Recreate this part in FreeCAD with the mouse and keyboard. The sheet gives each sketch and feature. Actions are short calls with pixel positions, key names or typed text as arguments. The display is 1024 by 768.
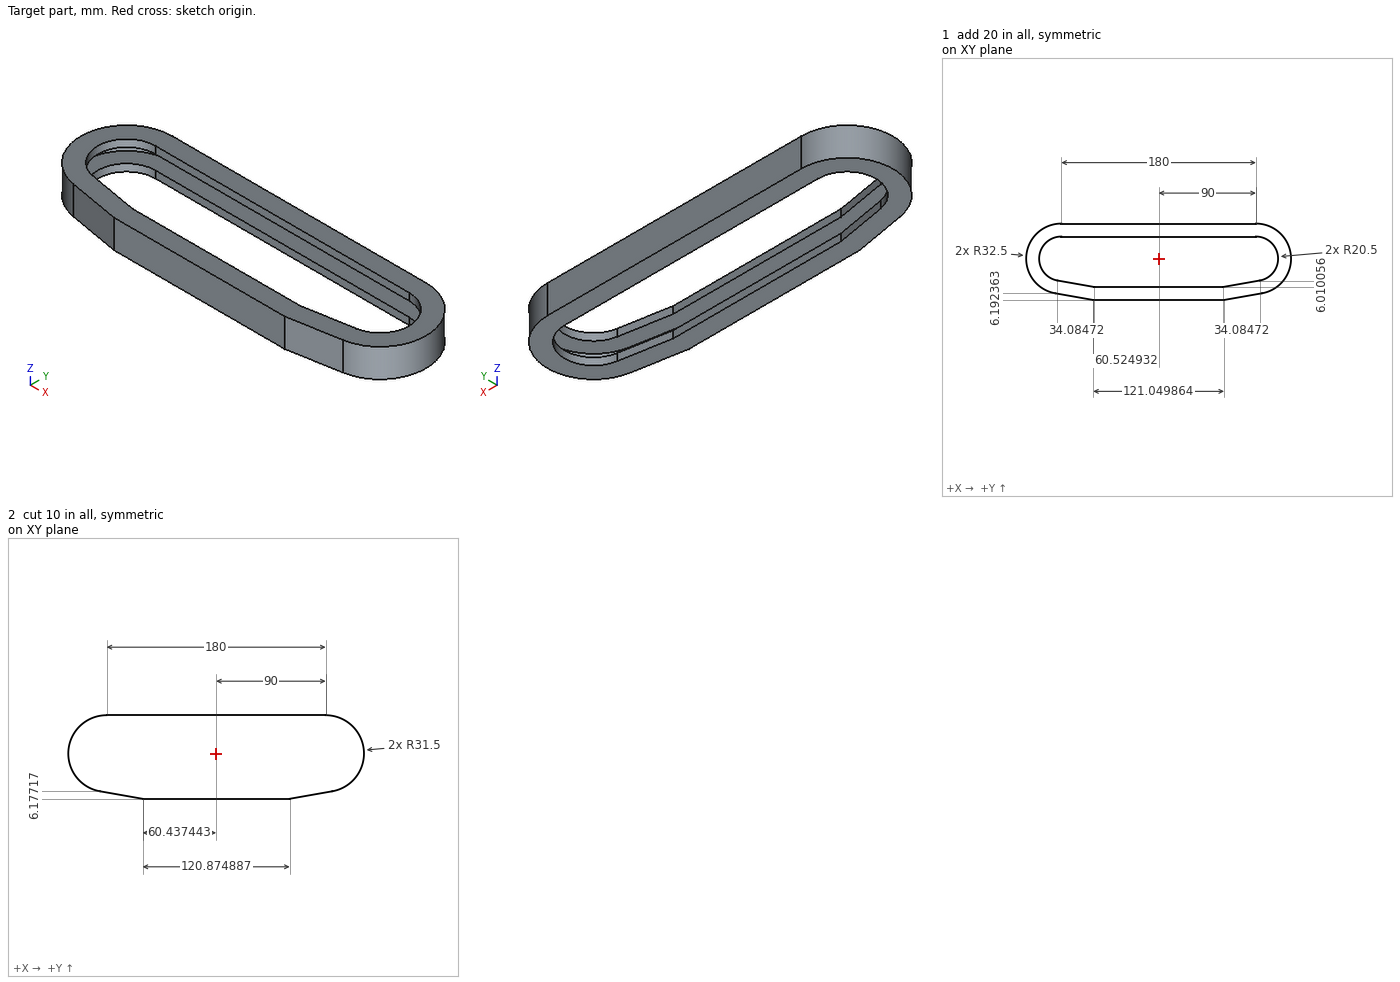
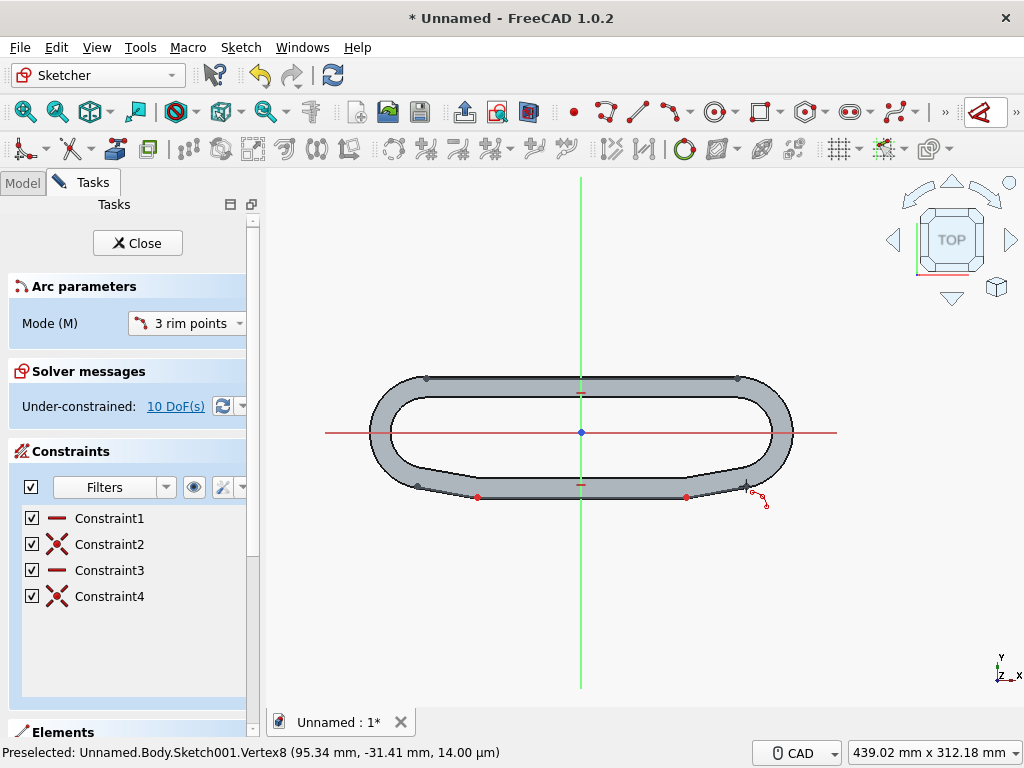
click(426, 379)
click(417, 487)
click(376, 412)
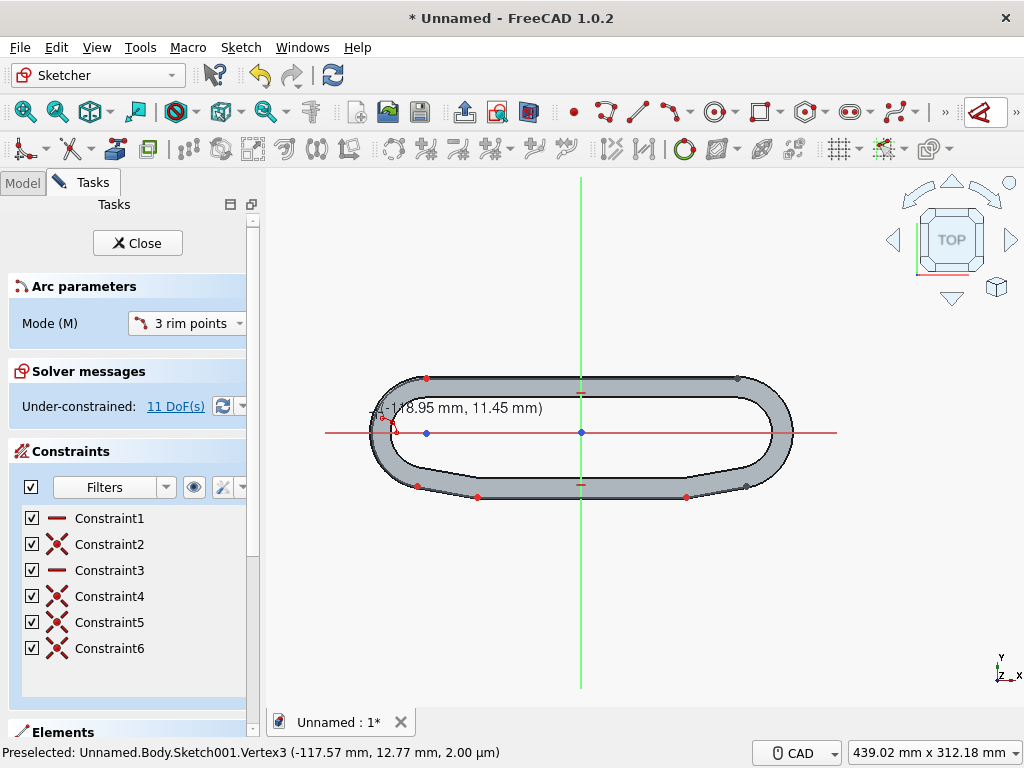
click(746, 487)
click(737, 379)
click(787, 412)
key(Escape)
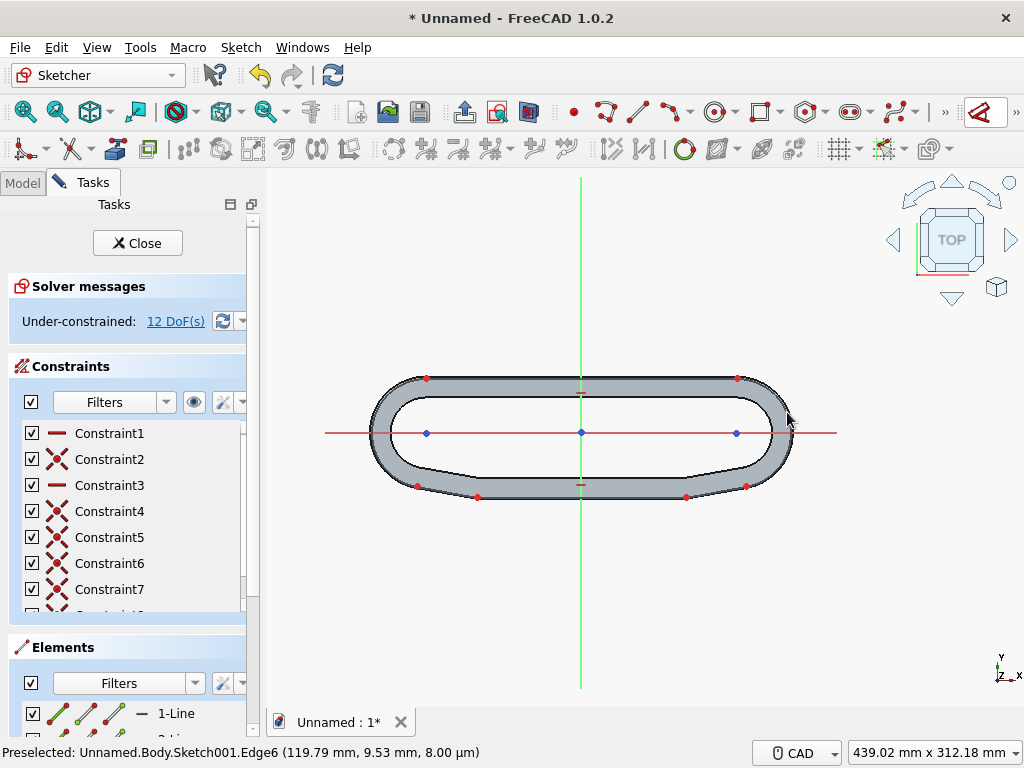
click(644, 379)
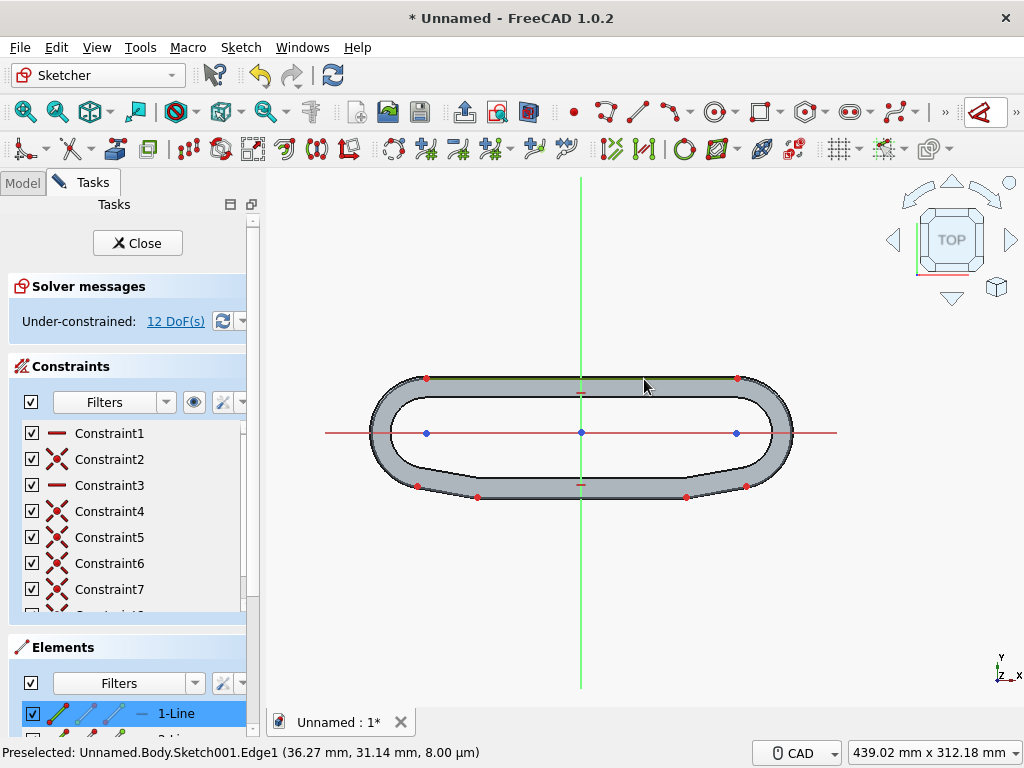
click(384, 399)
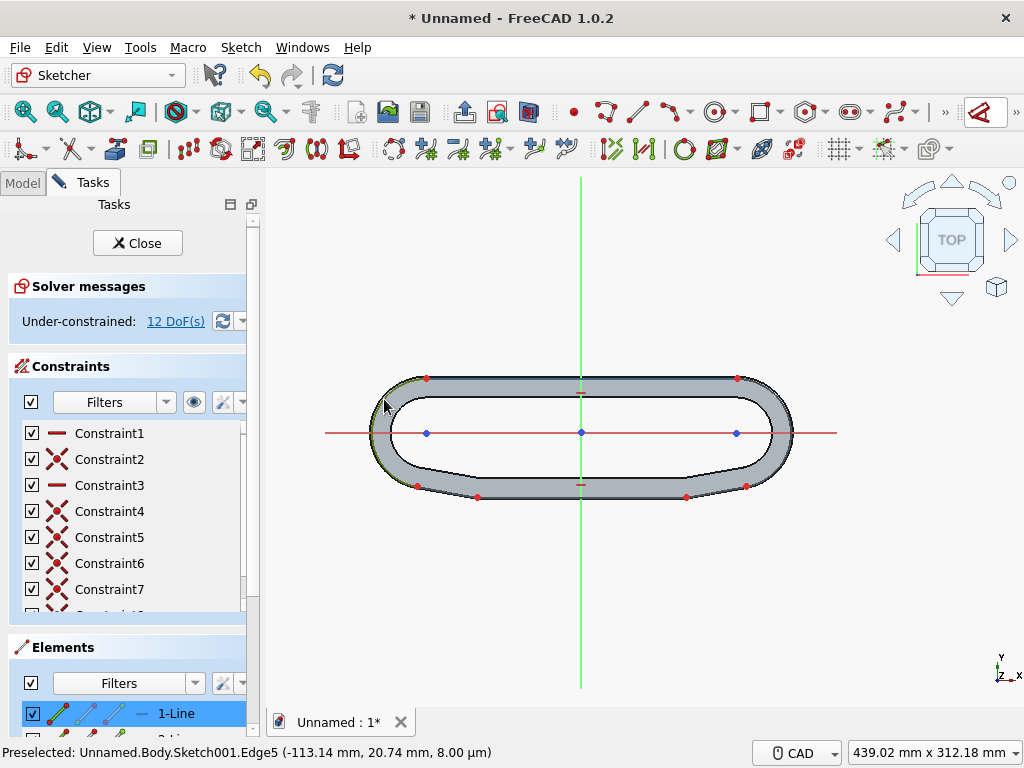
key(t)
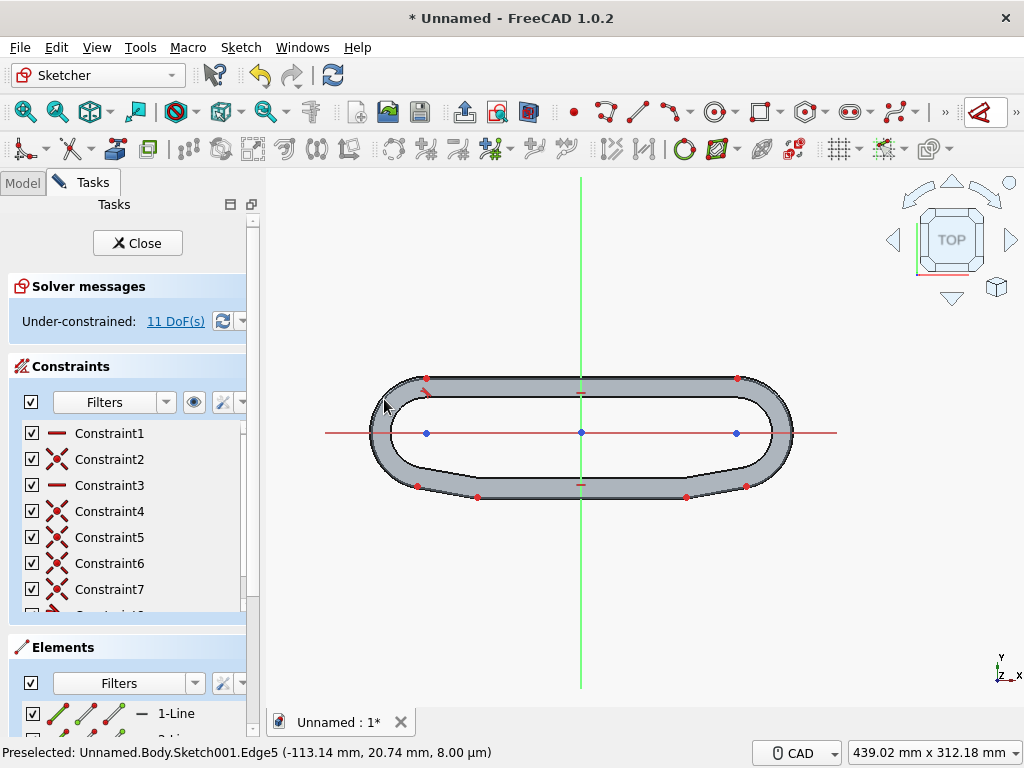
click(644, 379)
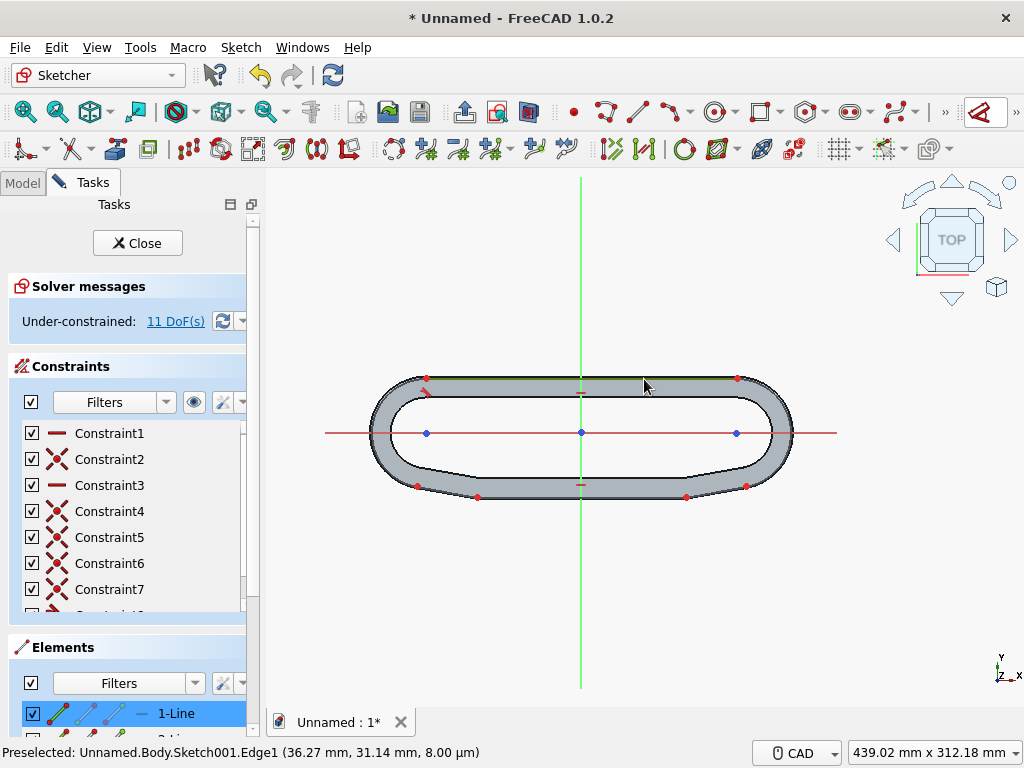
click(784, 460)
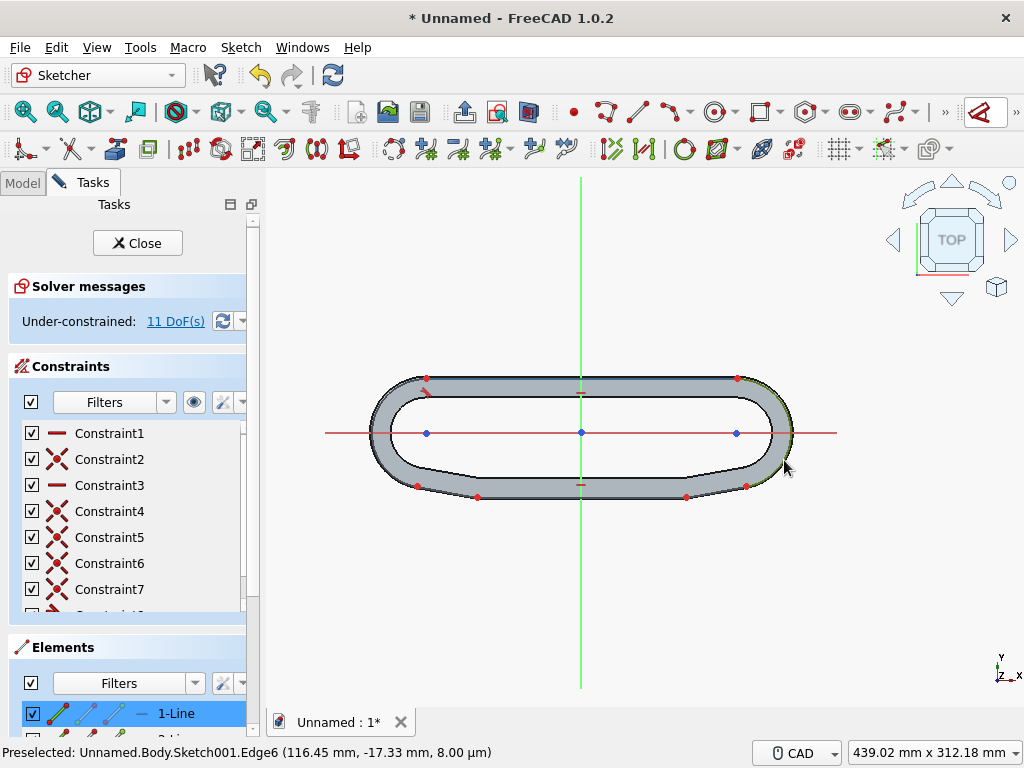
key(t)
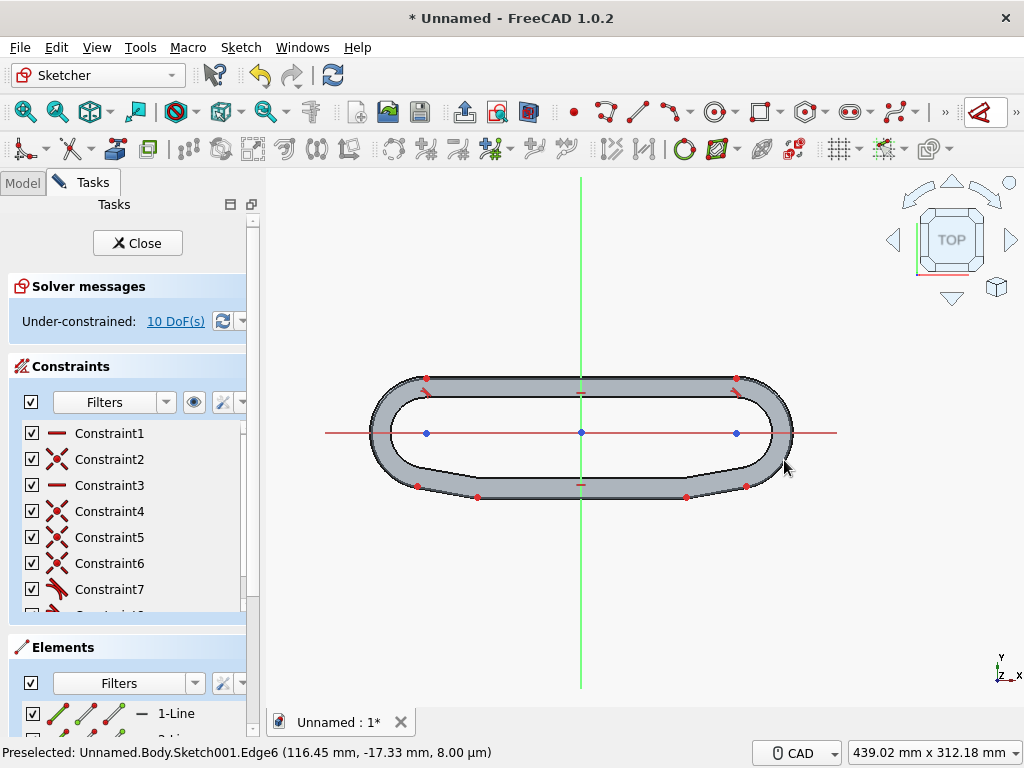
click(435, 490)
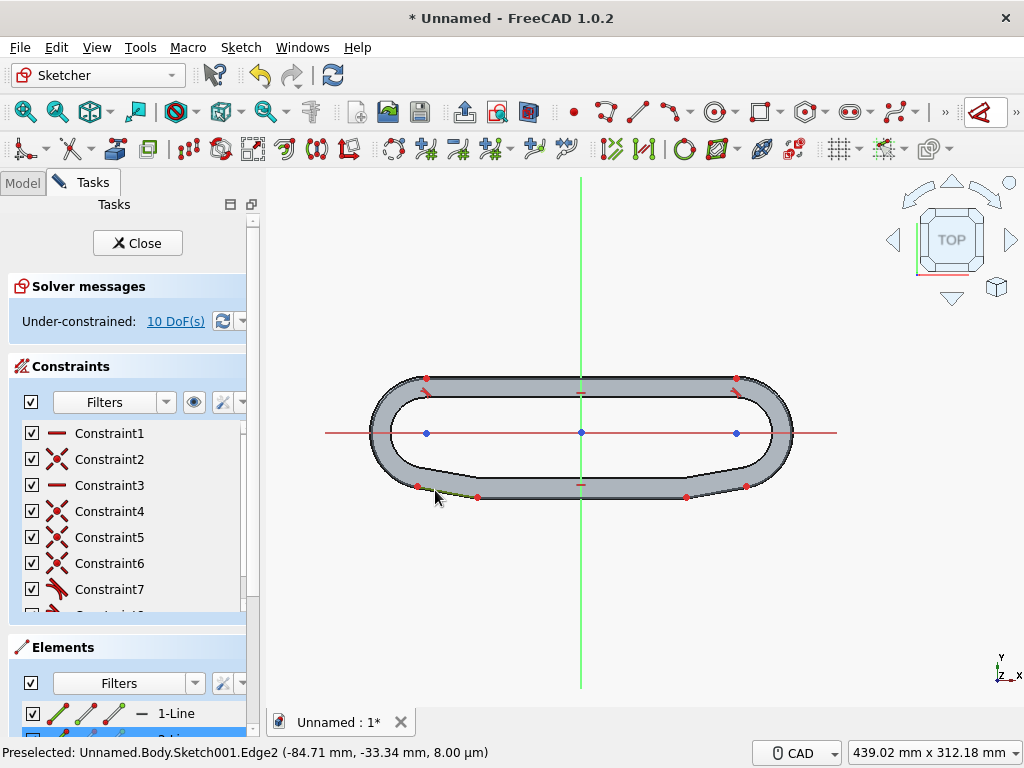
click(384, 399)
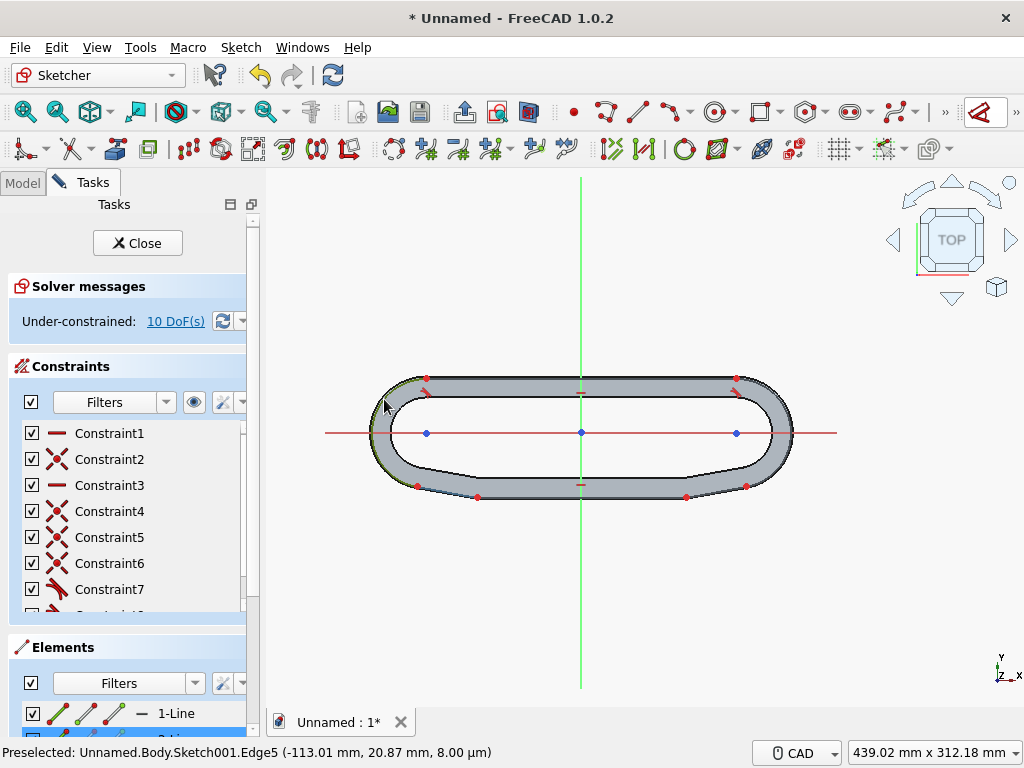
key(t)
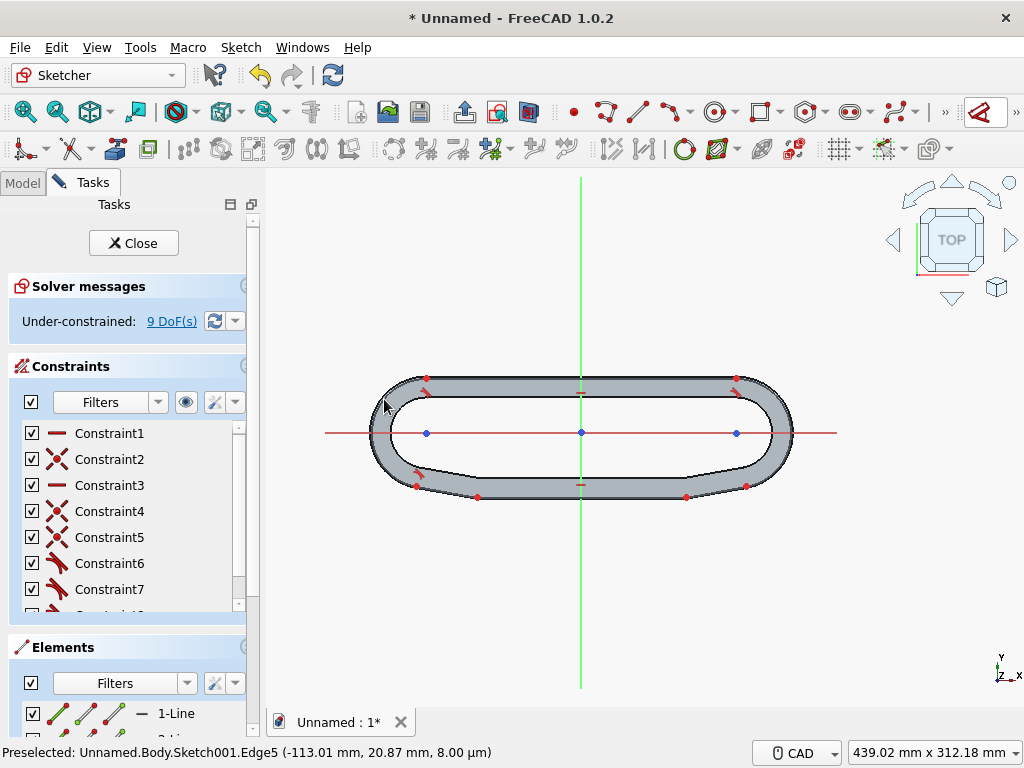
click(704, 495)